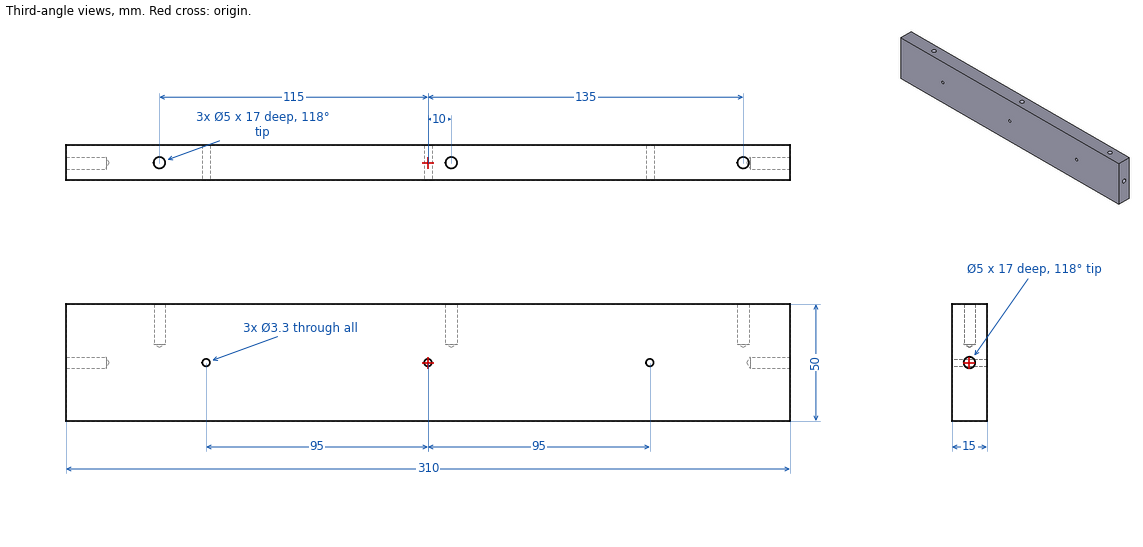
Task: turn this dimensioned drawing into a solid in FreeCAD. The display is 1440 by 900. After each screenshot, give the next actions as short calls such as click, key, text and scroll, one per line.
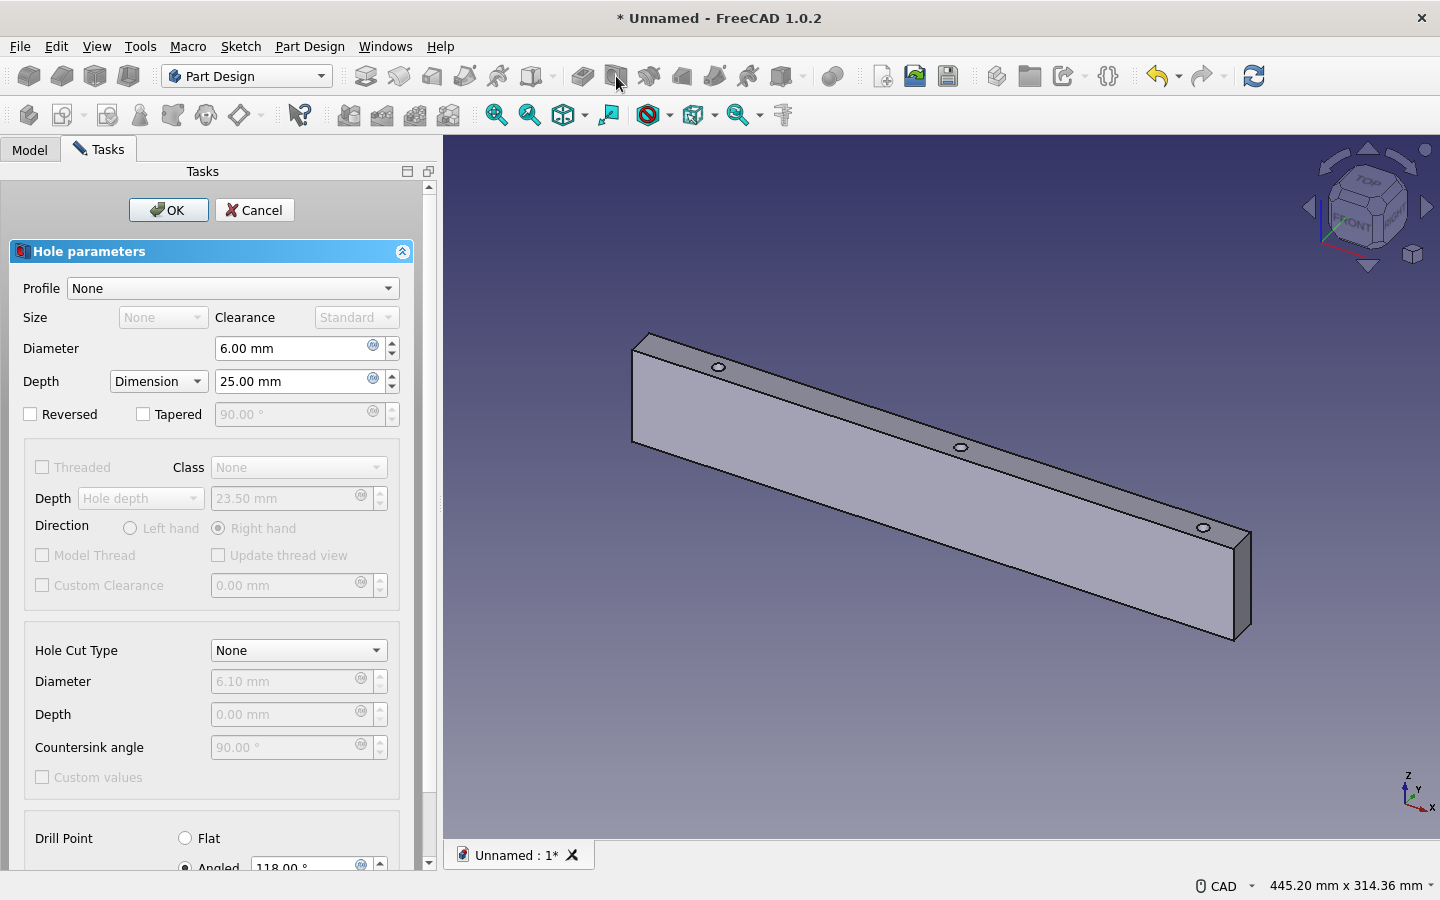
triple_click(300, 348)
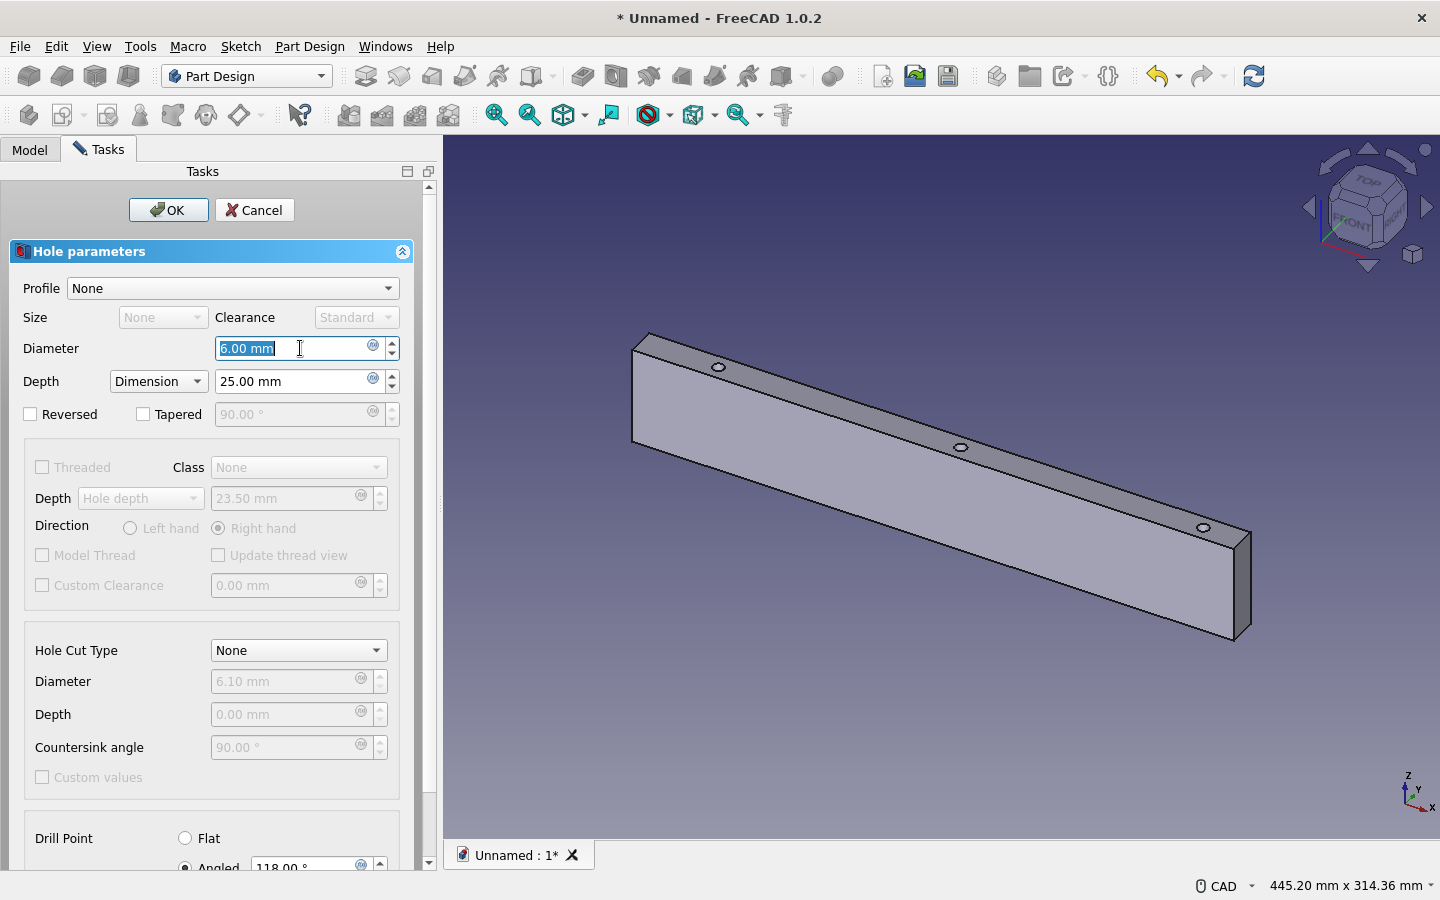
text(5)
key(Tab)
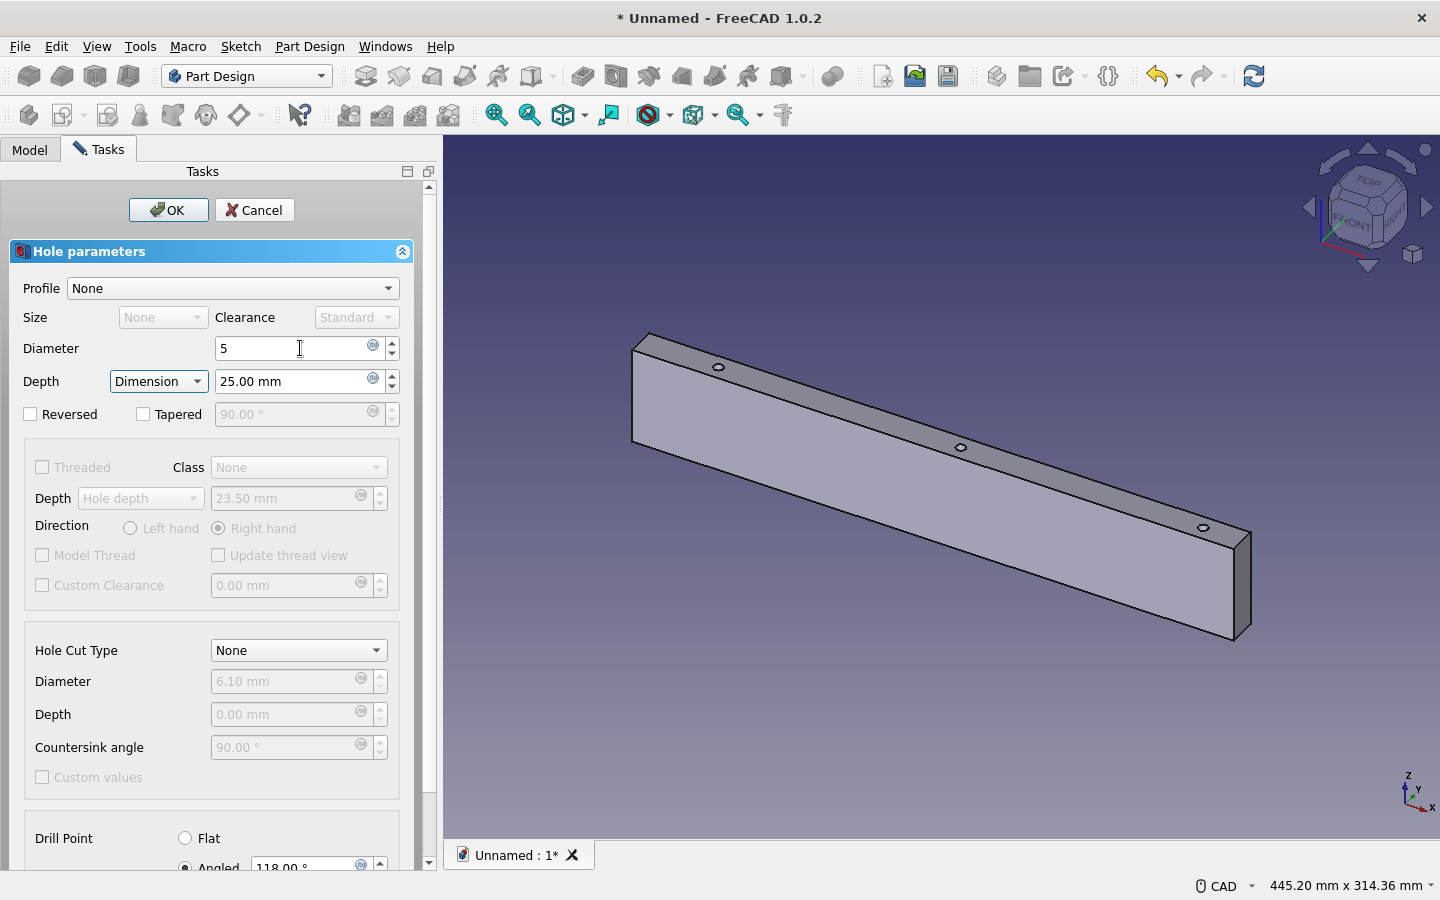
triple_click(300, 382)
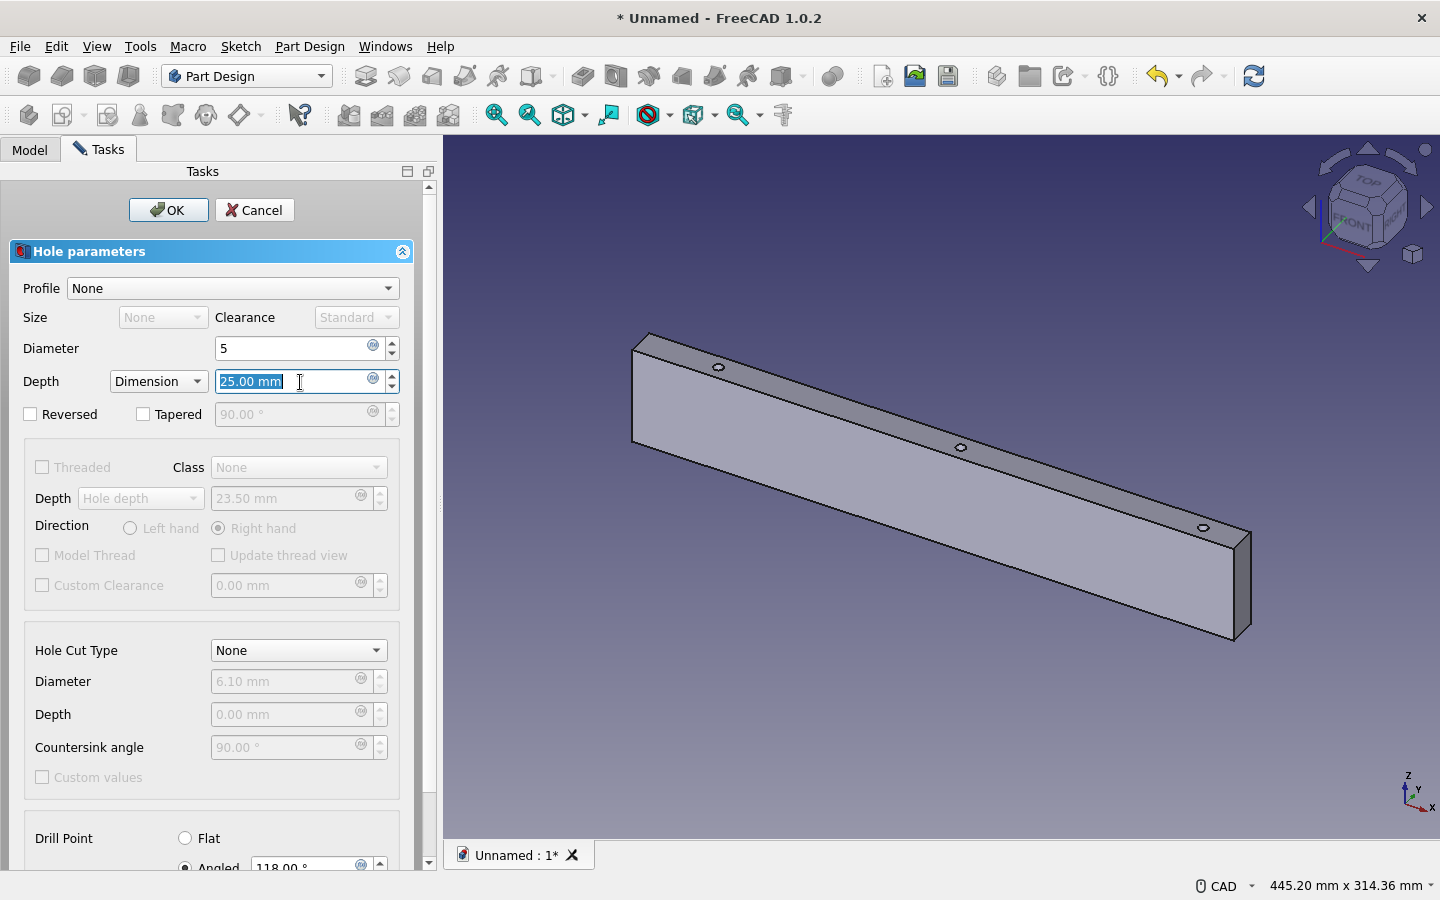
text(17)
key(Tab)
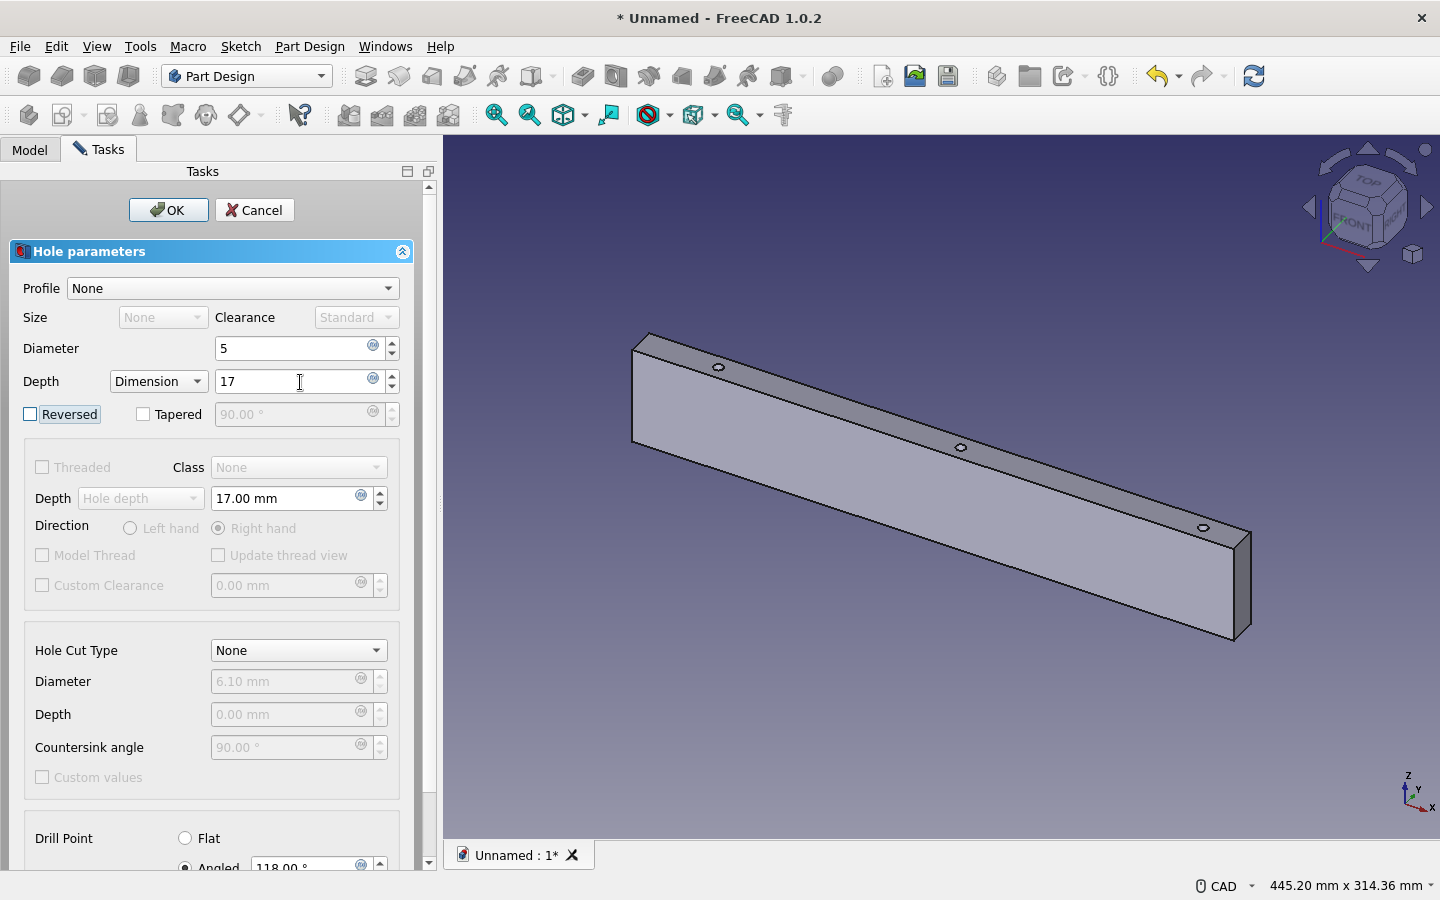
click(169, 210)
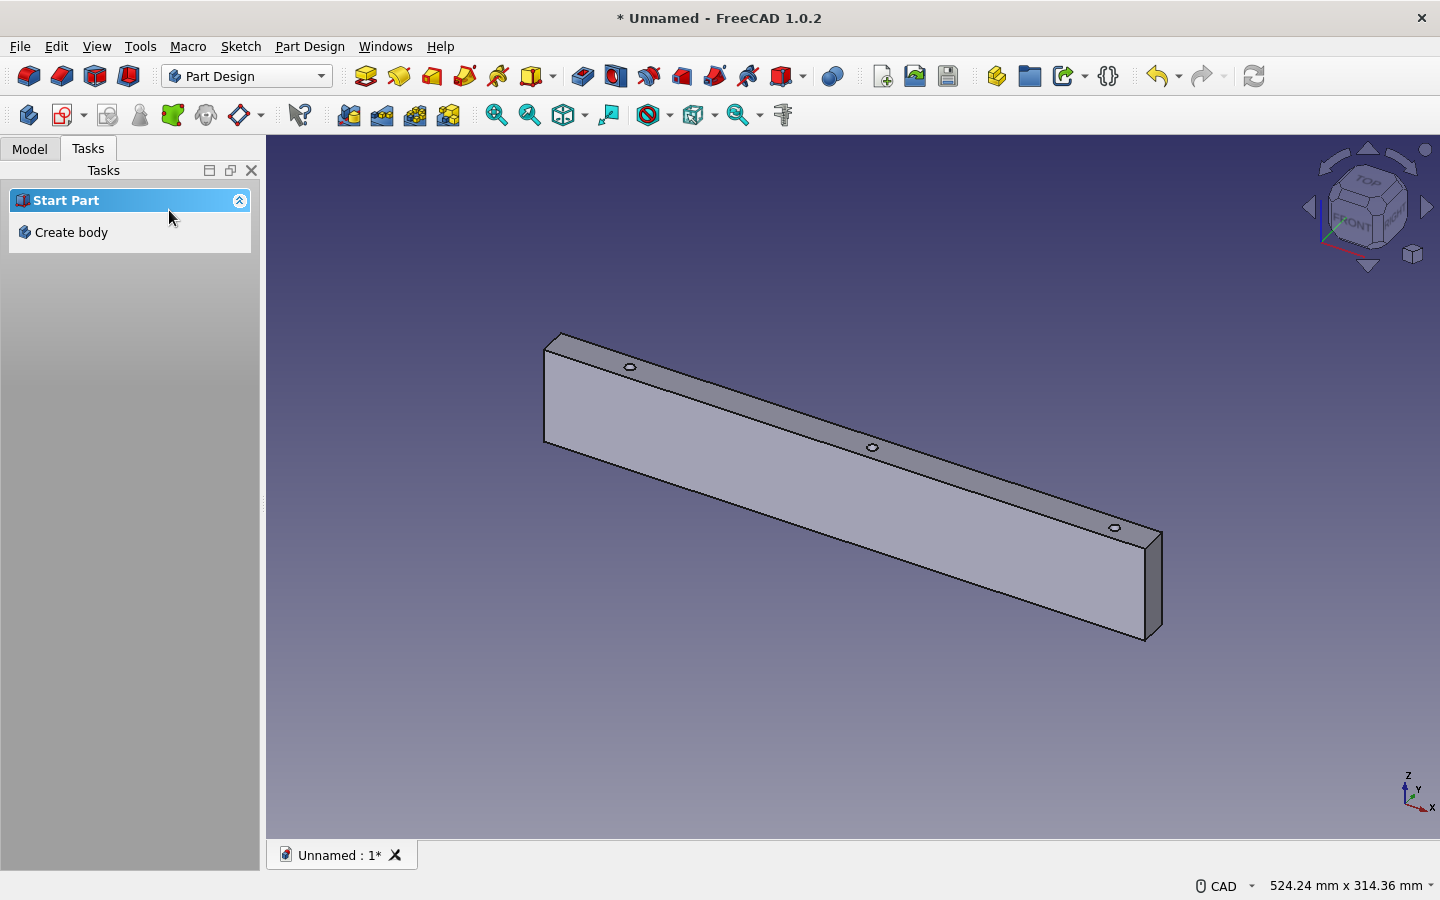
click(1154, 559)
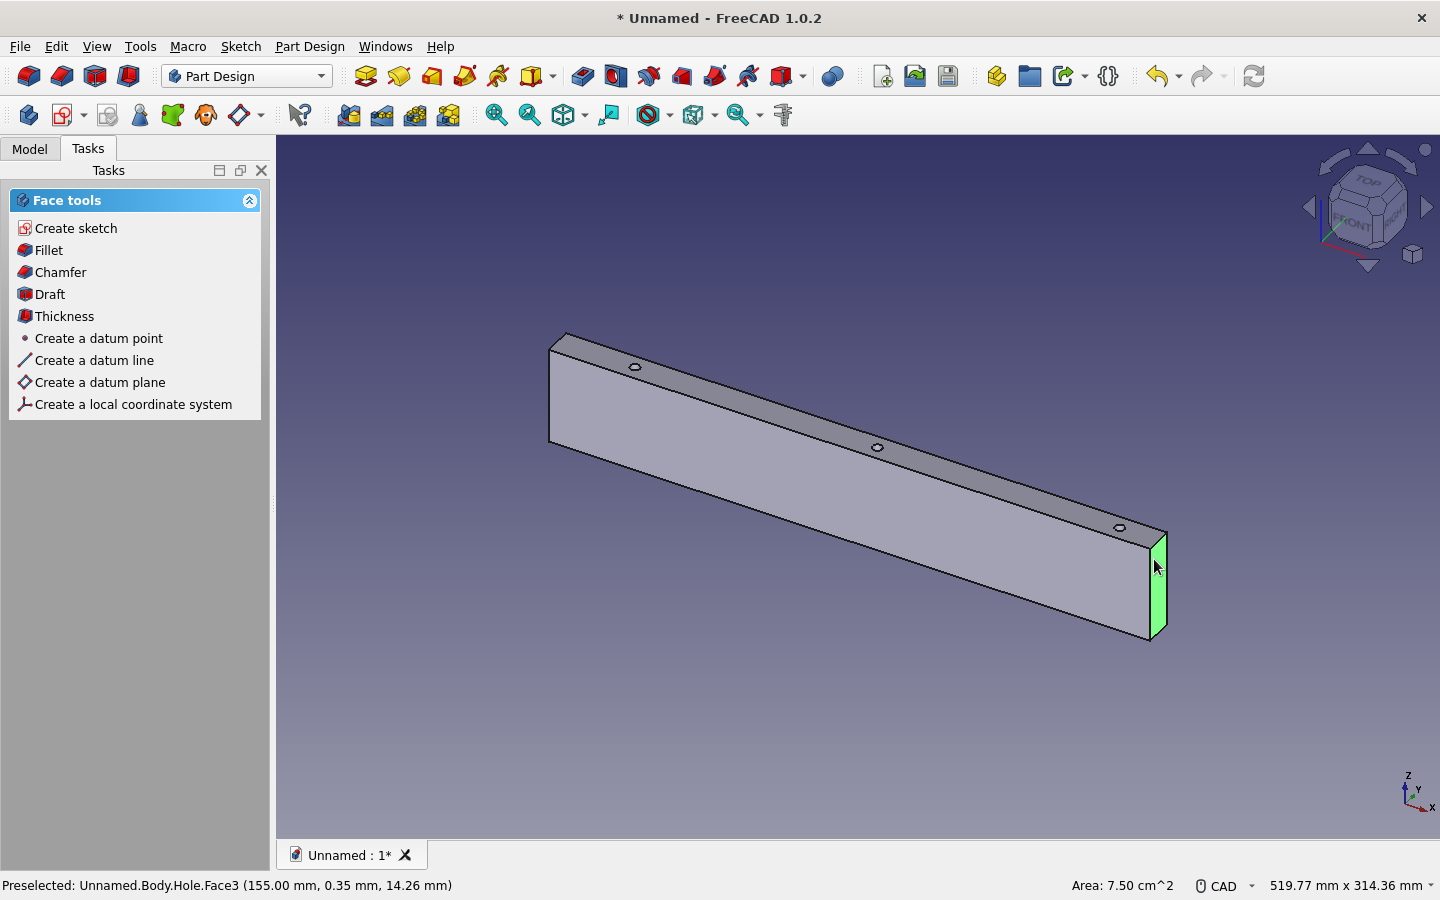
click(62, 116)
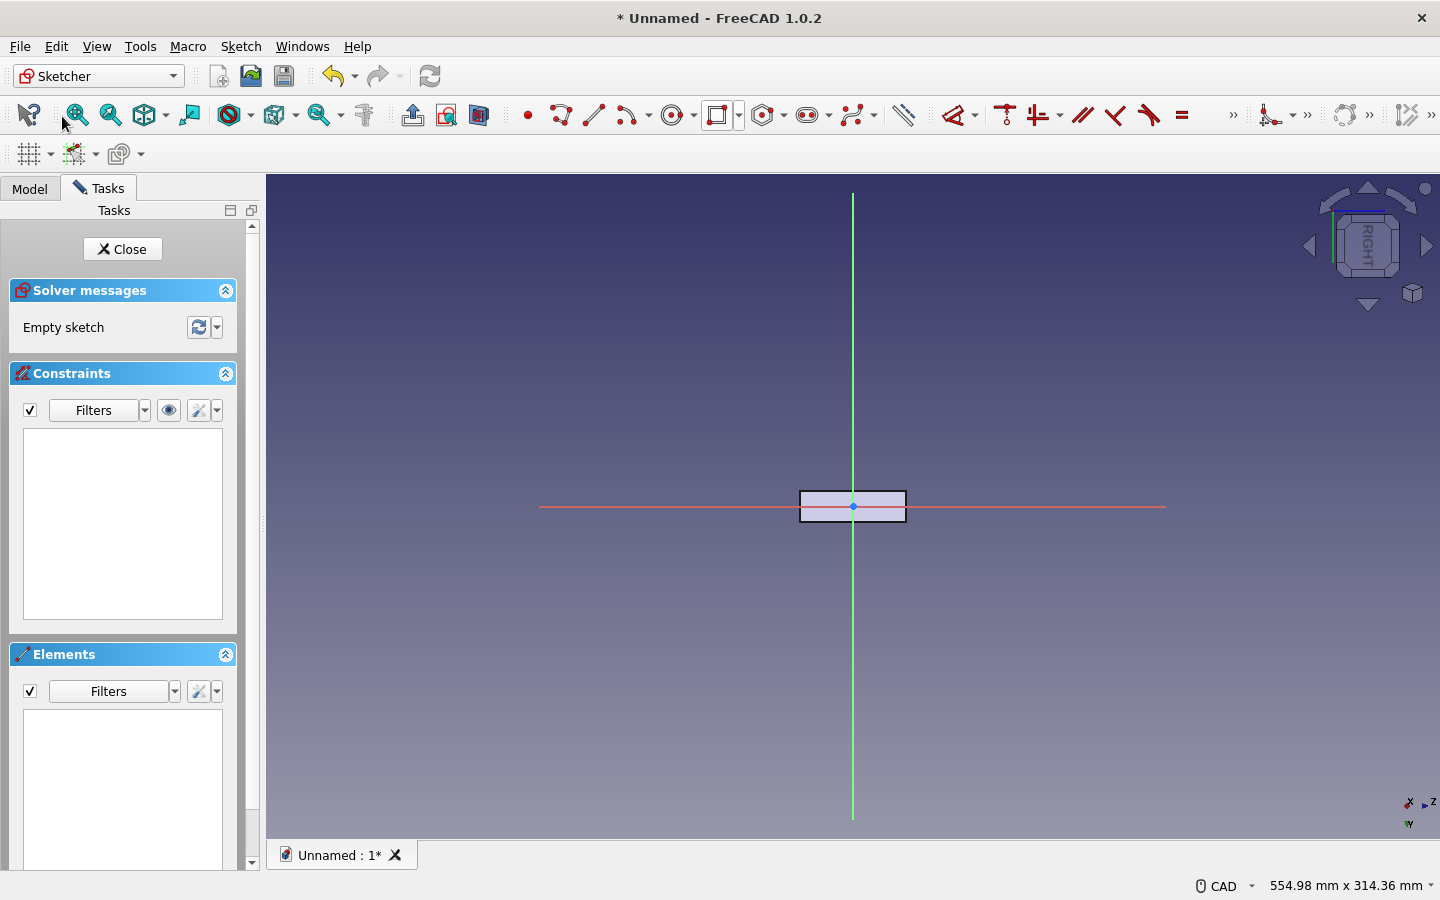
scroll(857, 506, up, 15)